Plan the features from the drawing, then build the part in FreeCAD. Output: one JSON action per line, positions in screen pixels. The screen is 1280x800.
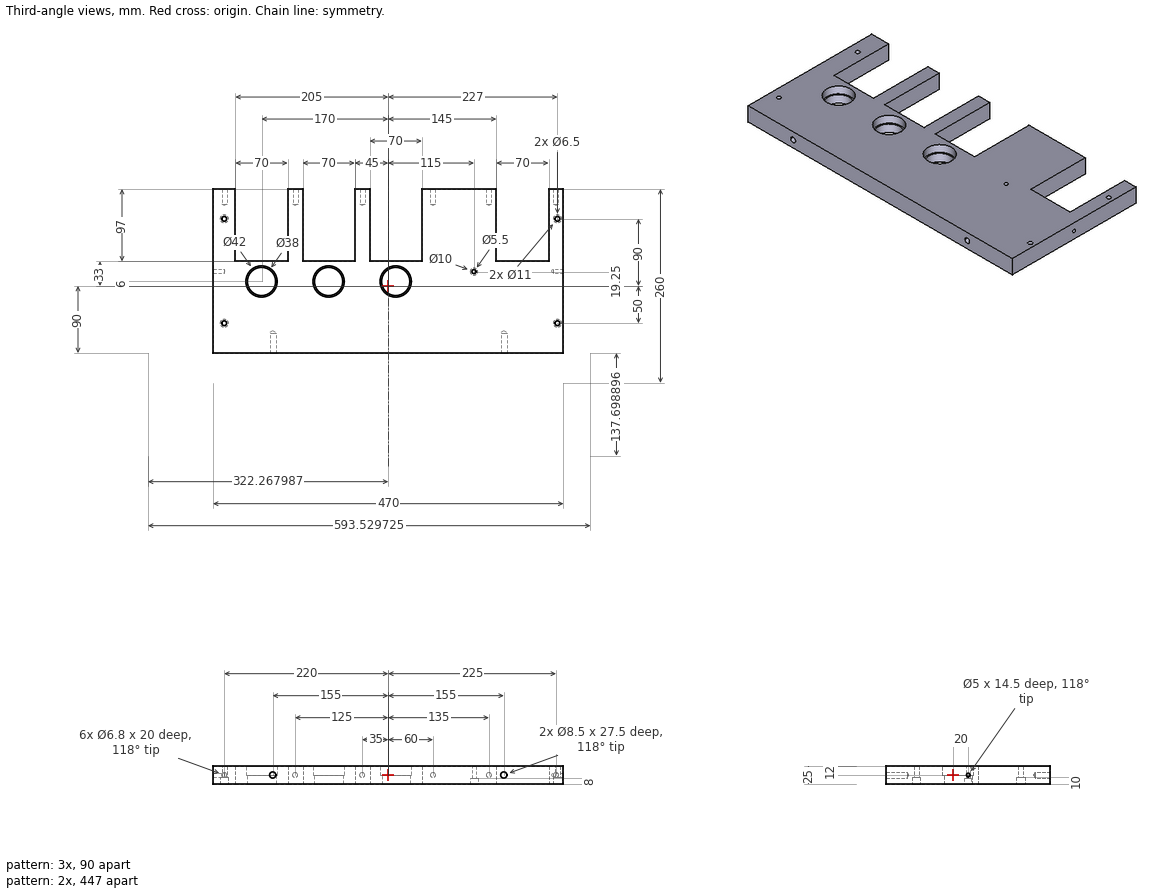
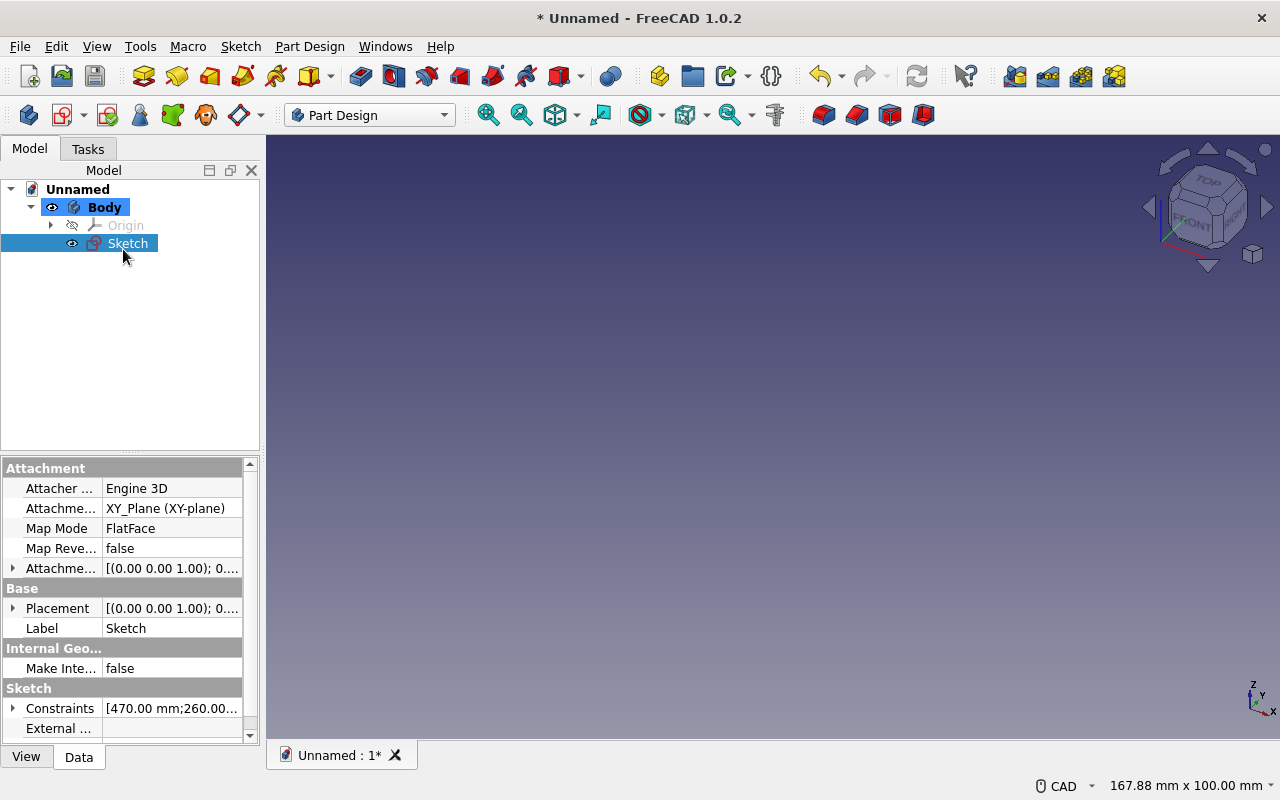
{"action": "left_click", "coordinate": [144, 76]}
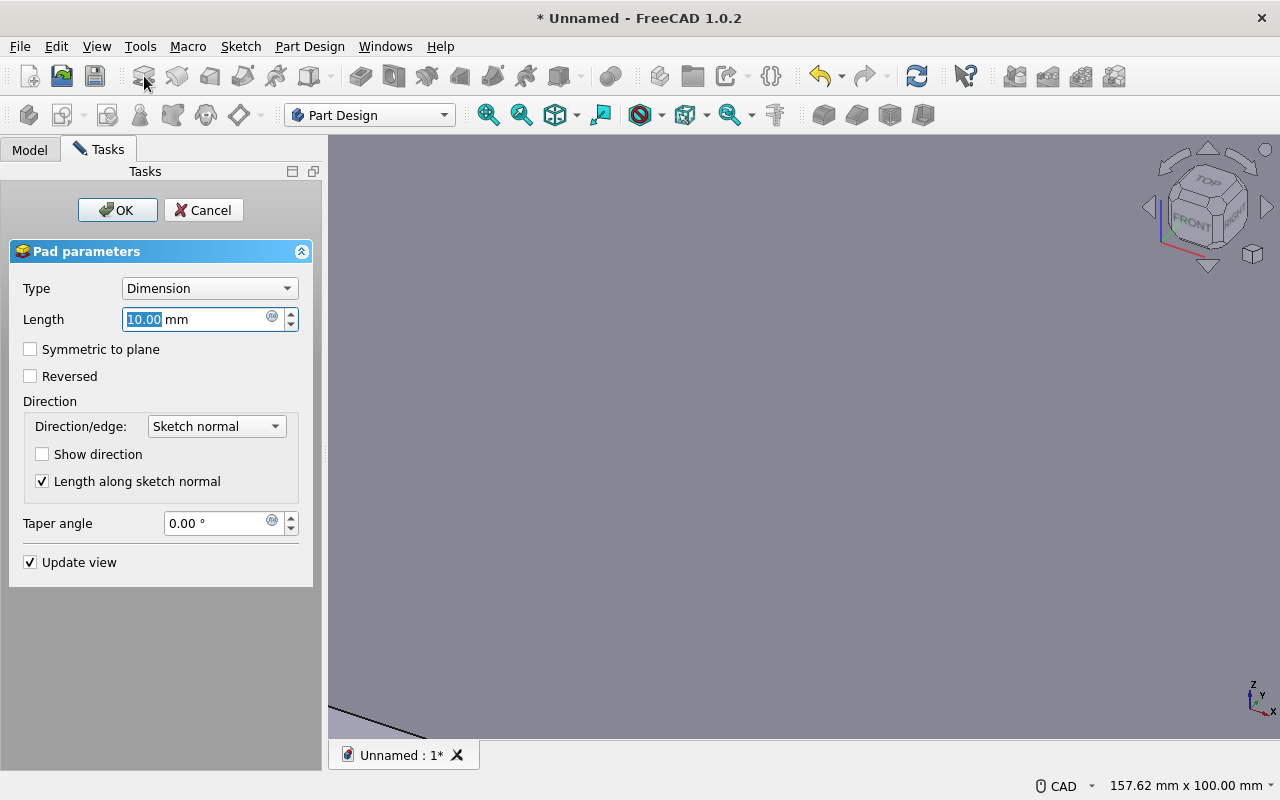
{"action": "type", "text": "25"}
{"action": "key", "text": "Tab"}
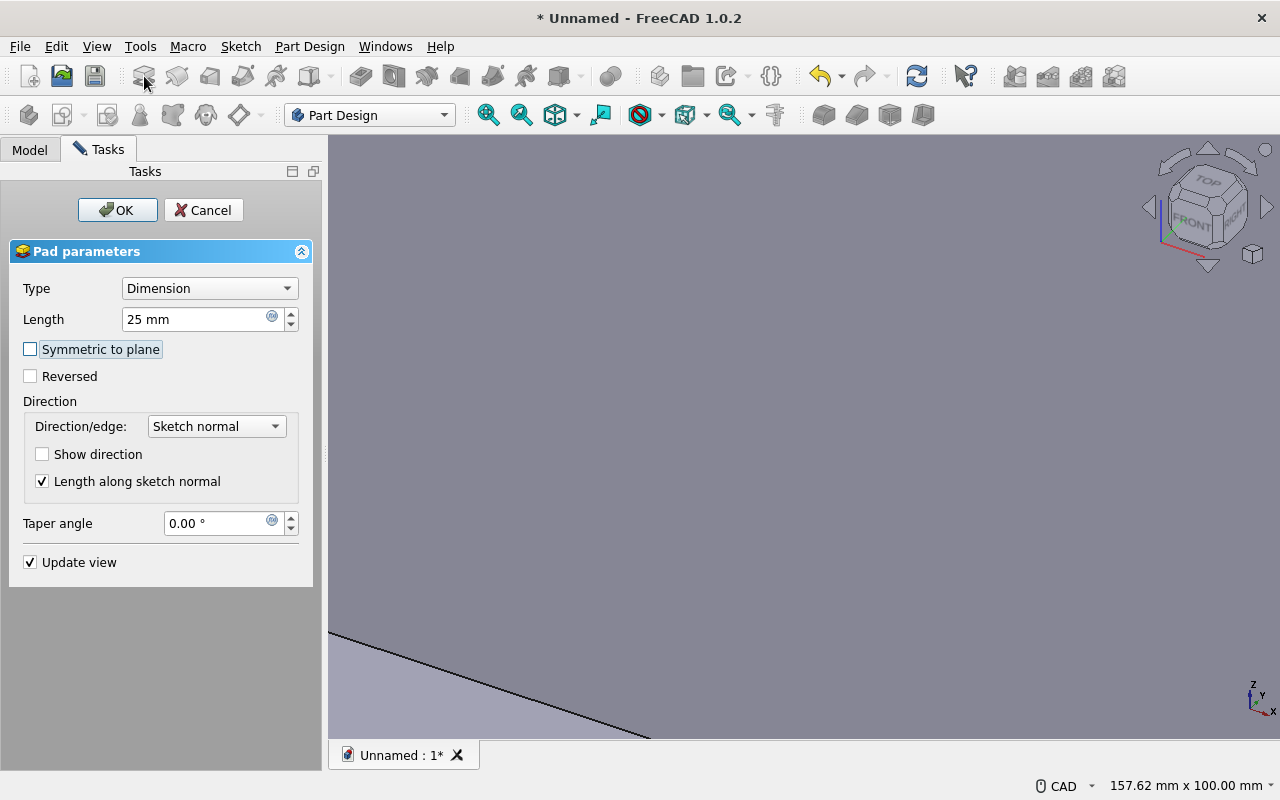
{"action": "left_click", "coordinate": [31, 349]}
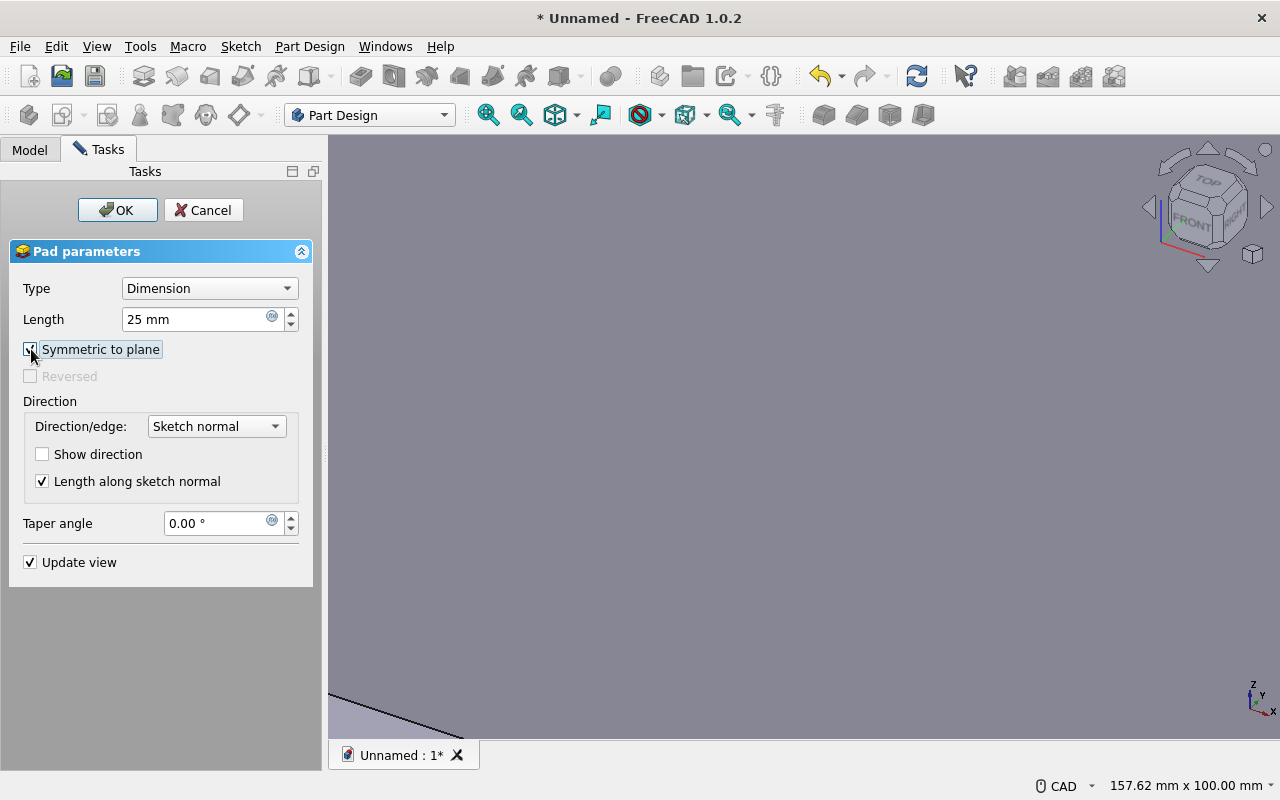
{"action": "left_click", "coordinate": [118, 210]}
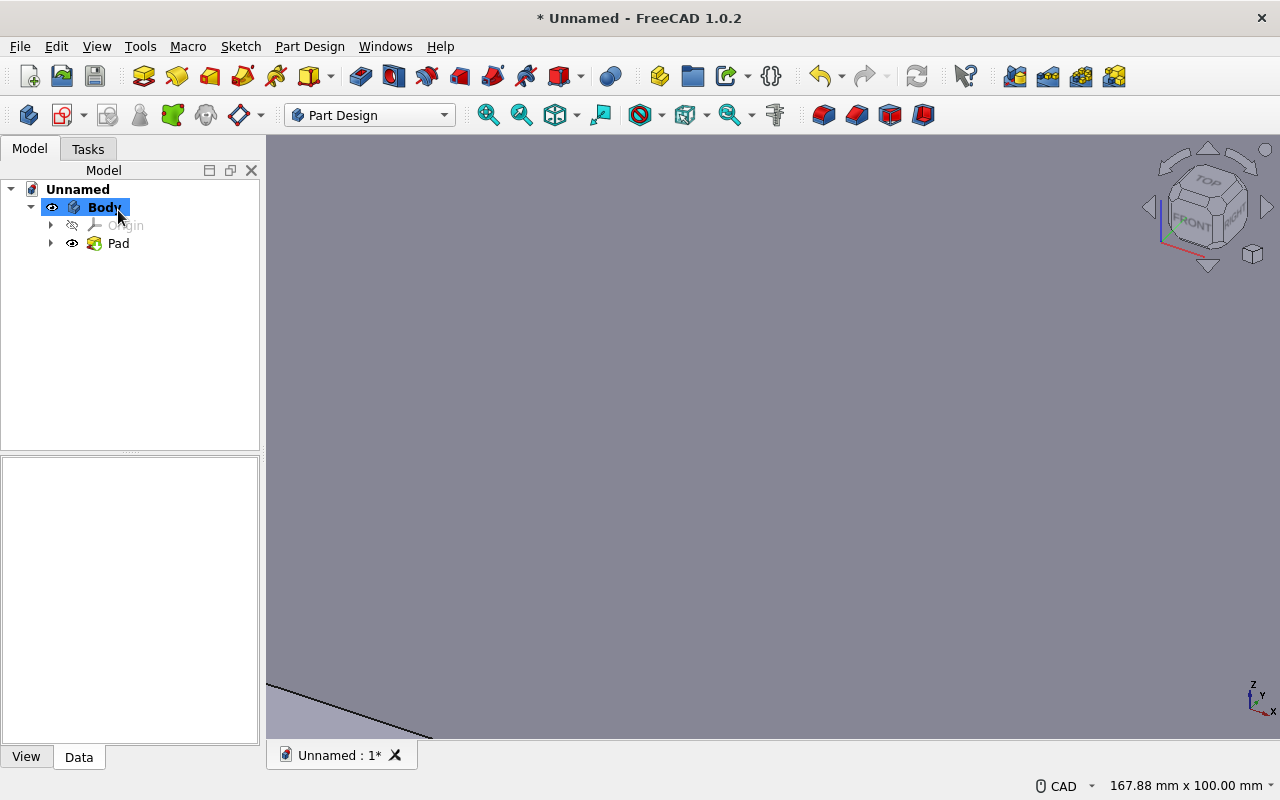
{"action": "left_click", "coordinate": [489, 116]}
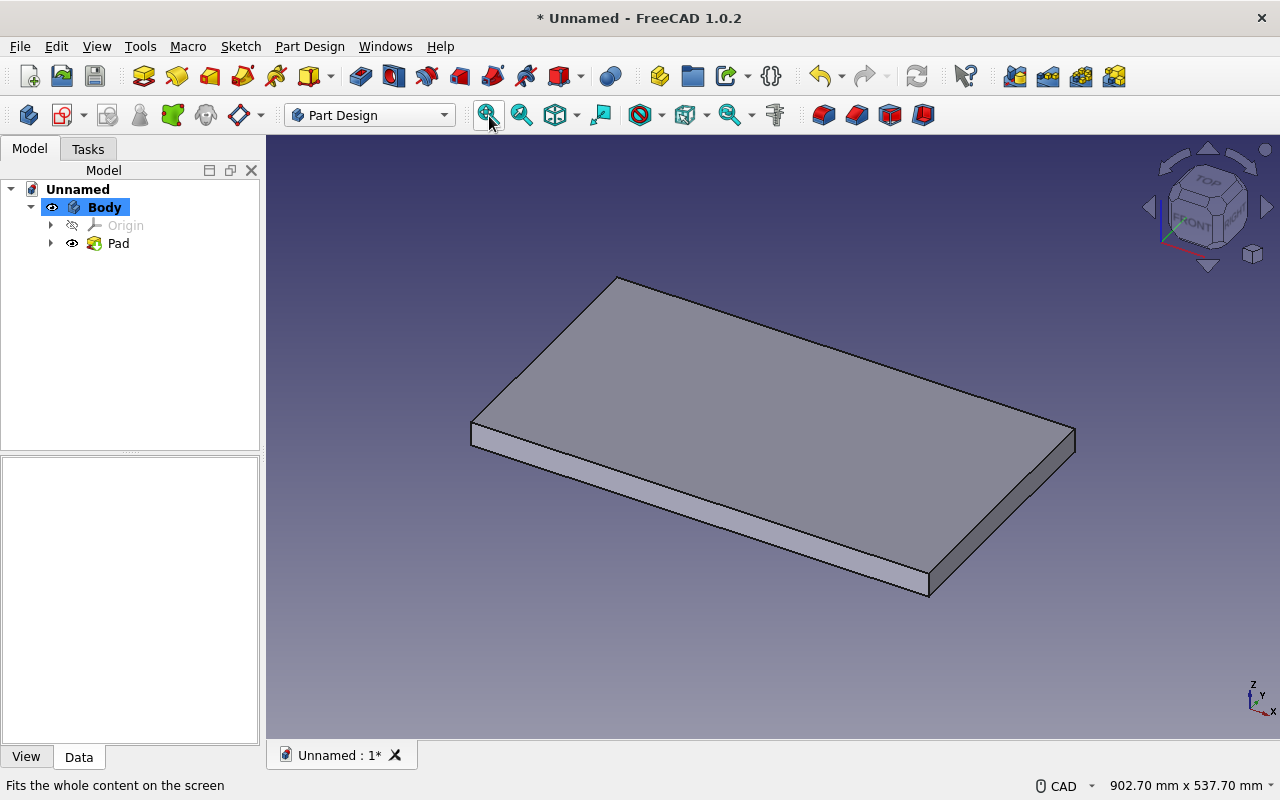
{"action": "left_click", "coordinate": [838, 446]}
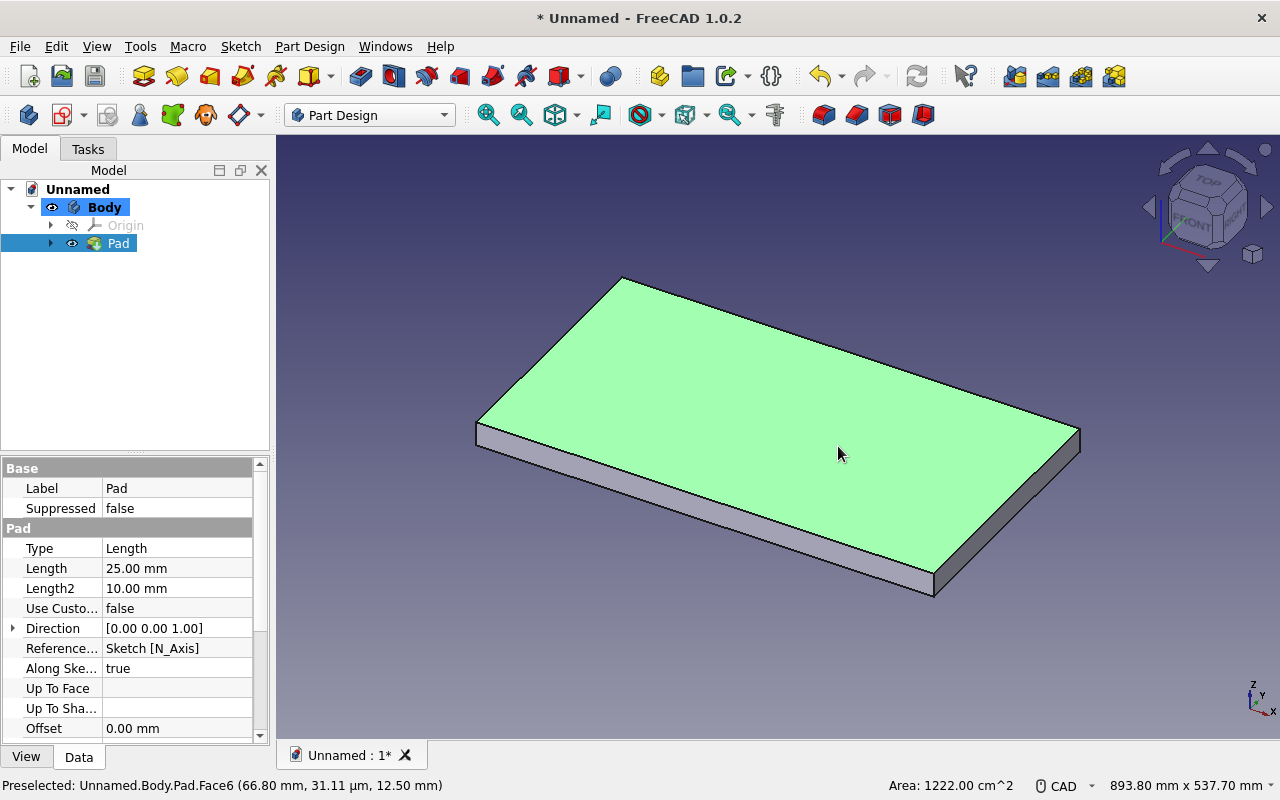
{"action": "left_click", "coordinate": [62, 116]}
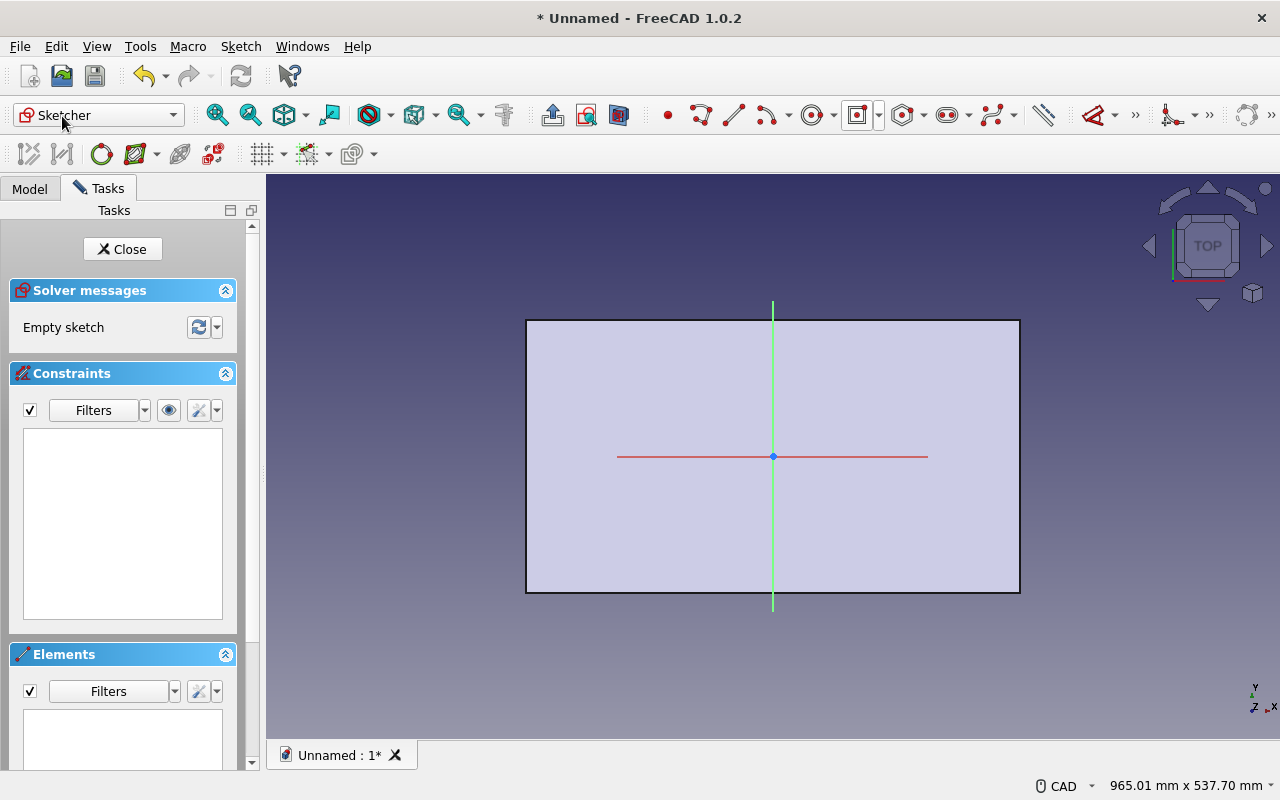
{"action": "key", "text": "g r"}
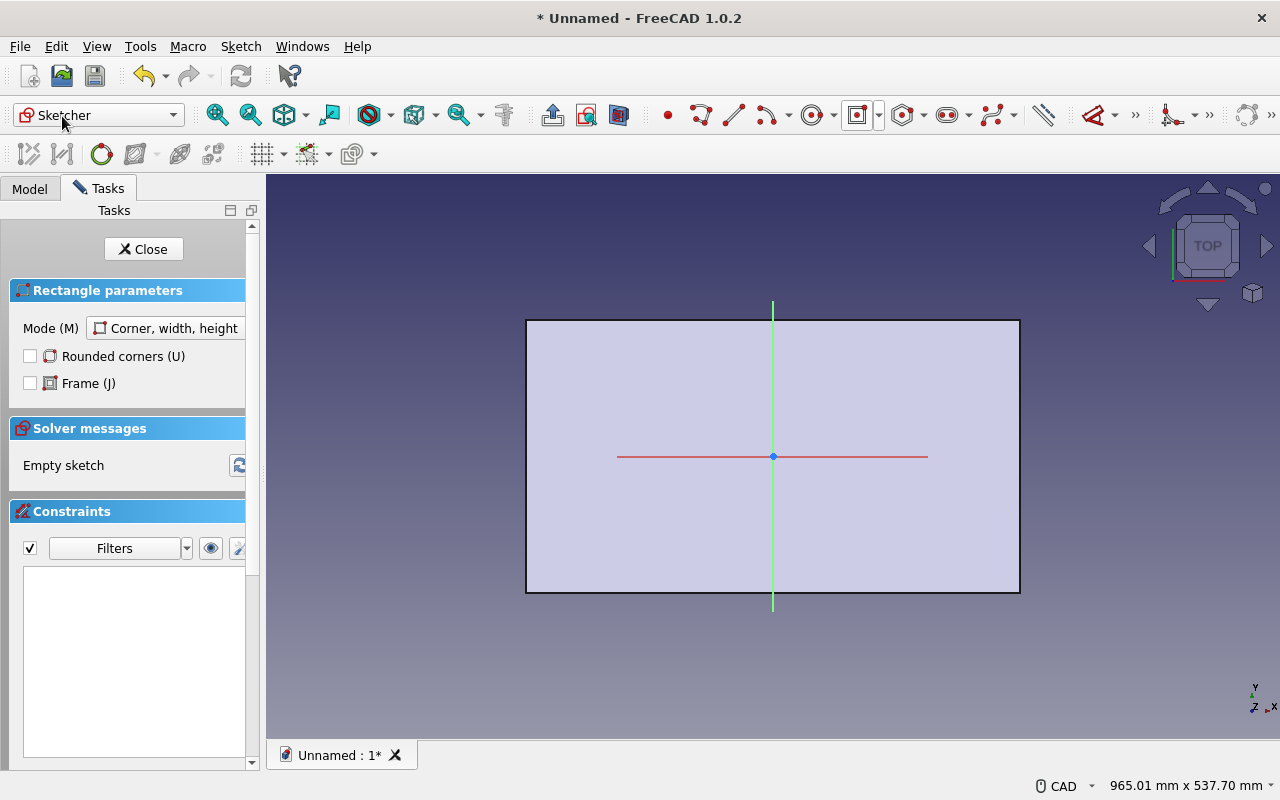
{"action": "left_click", "coordinate": [558, 320]}
{"action": "mouse_move", "coordinate": [631, 422]}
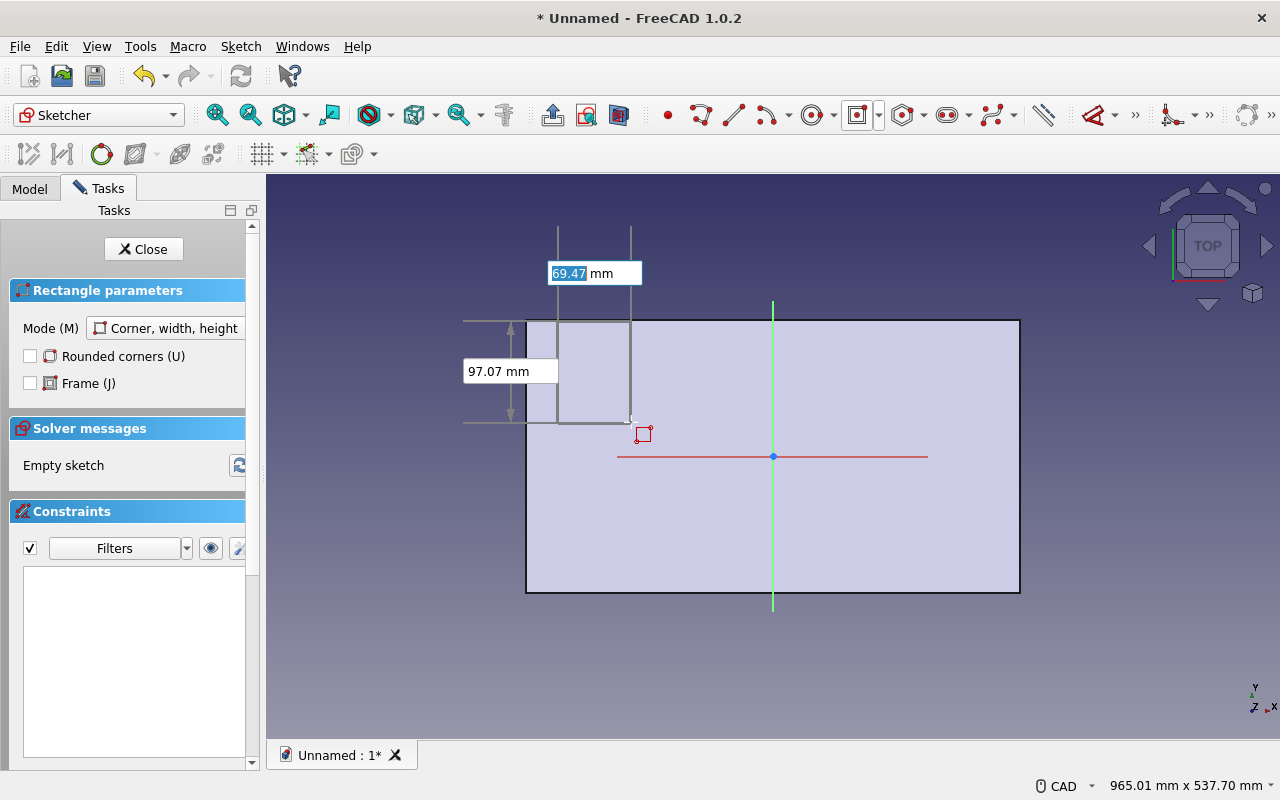
{"action": "type", "text": "70"}
{"action": "key", "text": "Tab"}
{"action": "type", "text": "97"}
{"action": "key", "text": "Return"}